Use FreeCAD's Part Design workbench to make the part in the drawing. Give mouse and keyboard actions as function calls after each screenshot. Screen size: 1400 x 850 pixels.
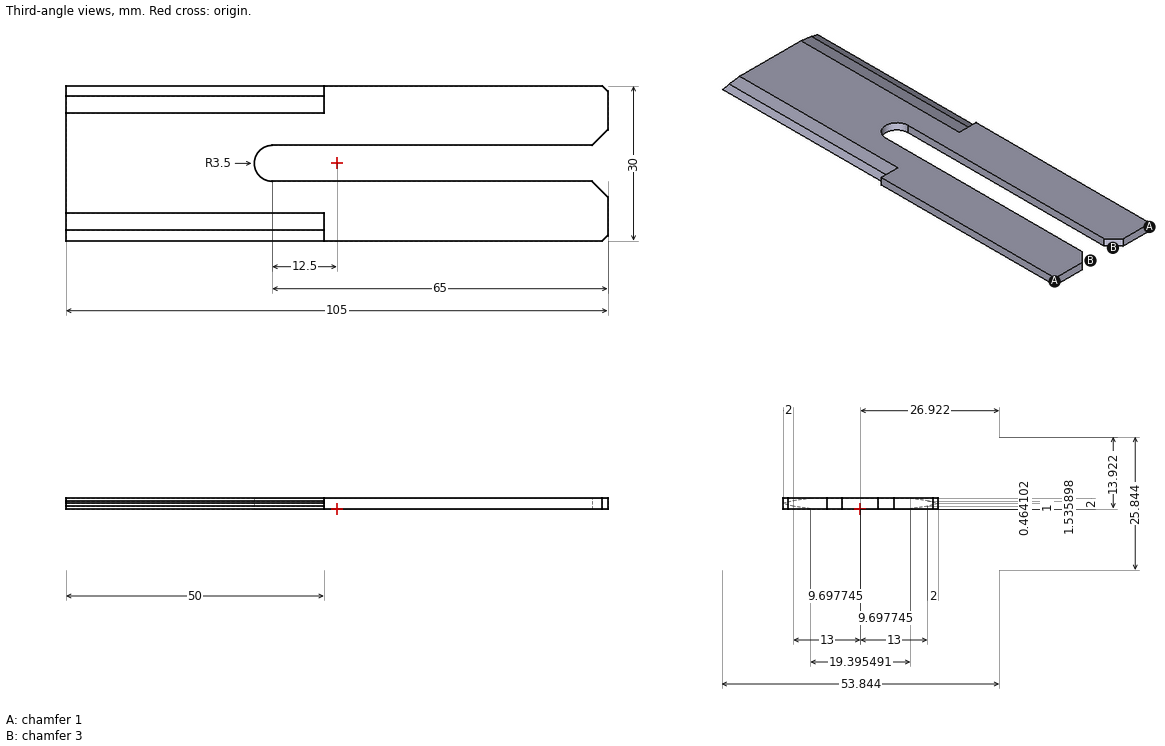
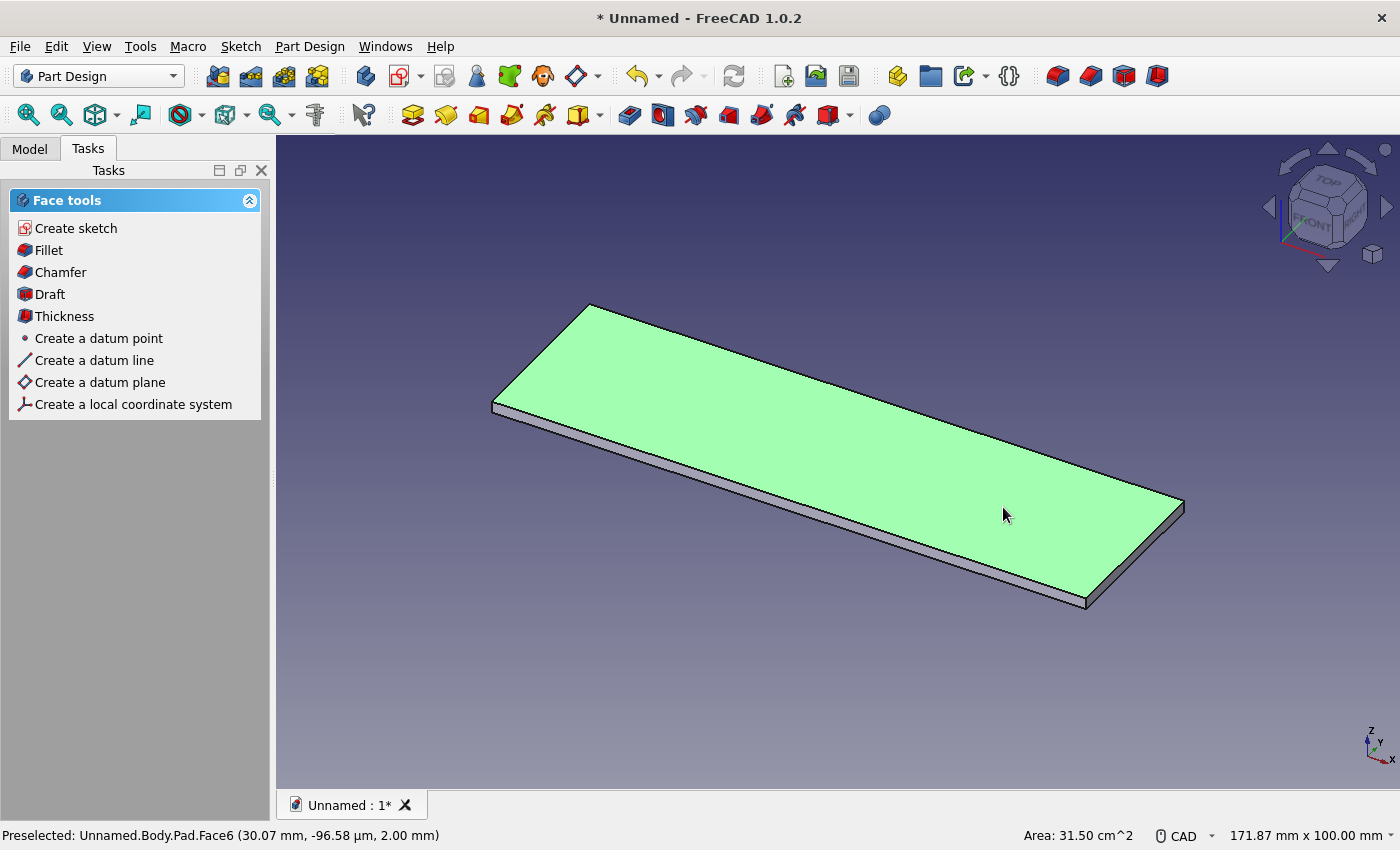
click(398, 76)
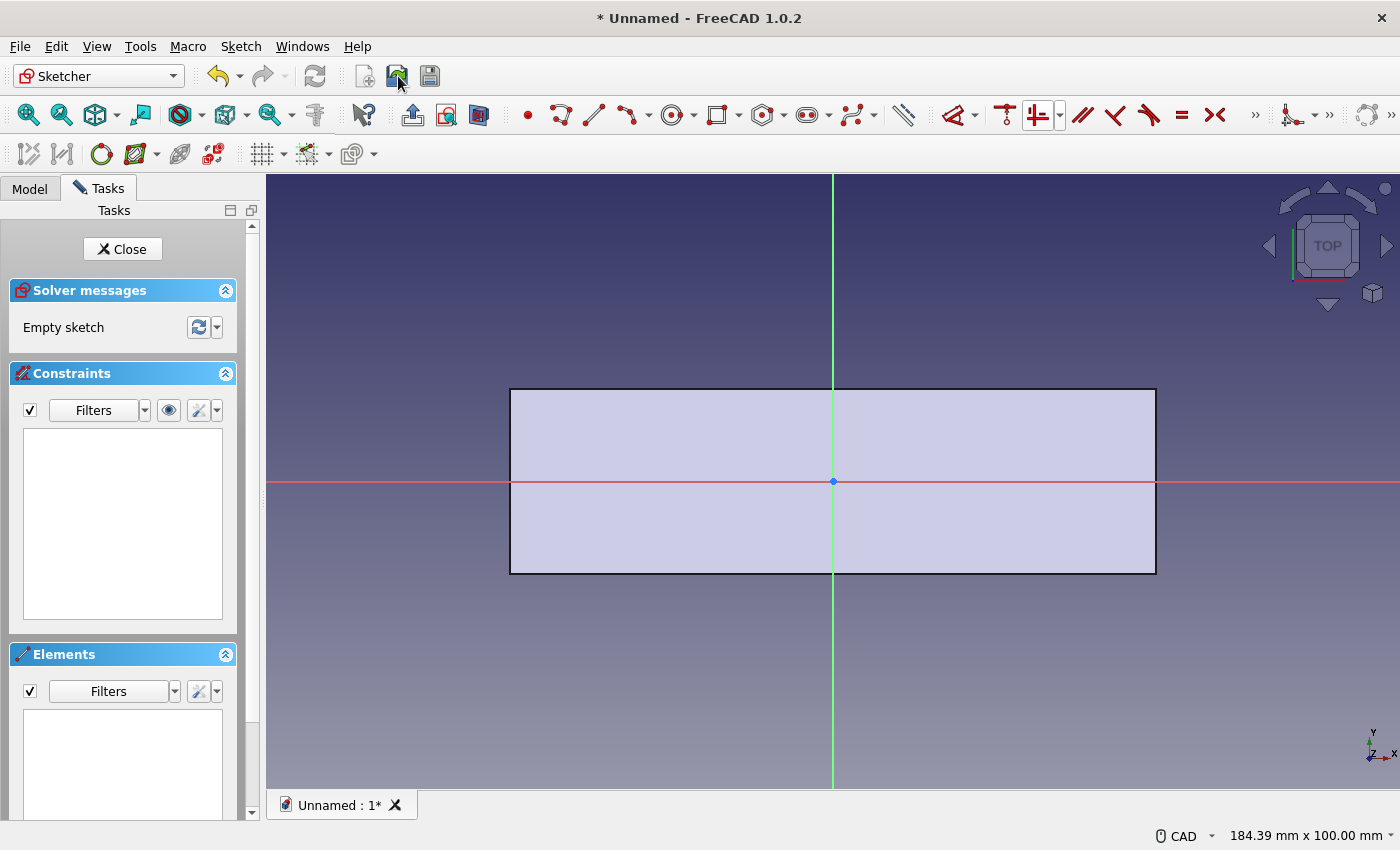
scroll(1235, 482, up, 2)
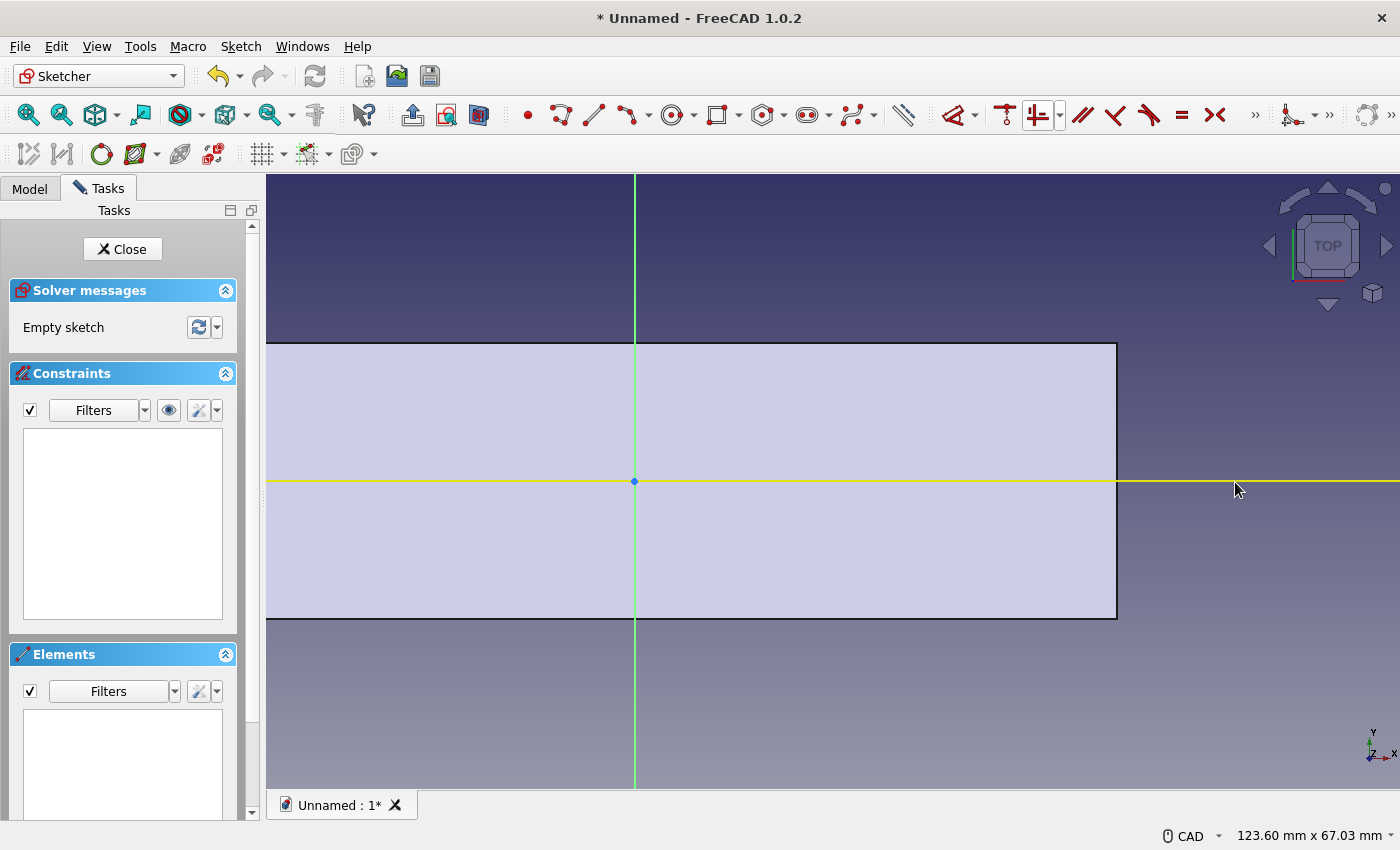
click(561, 116)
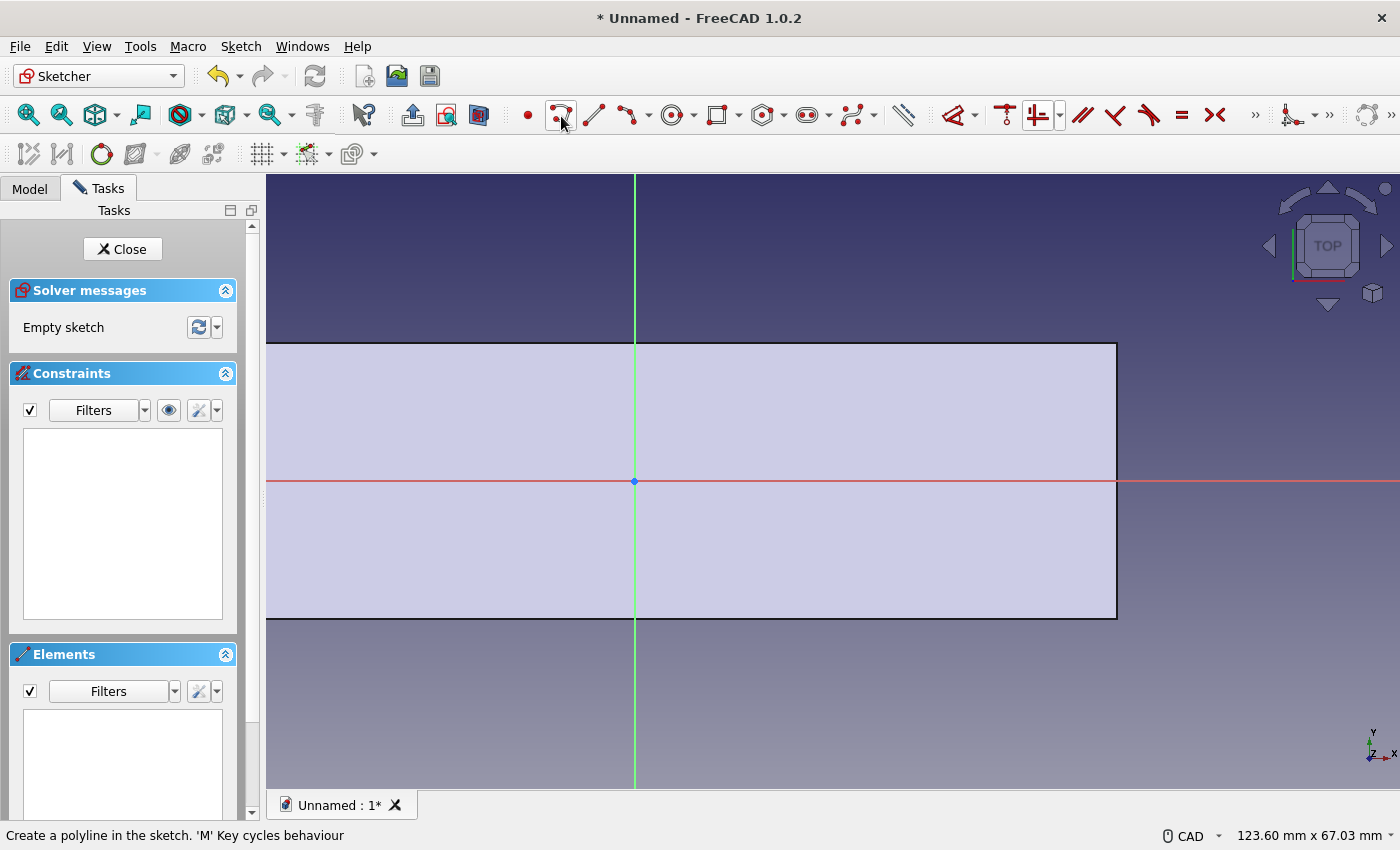
click(520, 513)
click(1117, 513)
click(1117, 449)
click(520, 449)
right_click(520, 449)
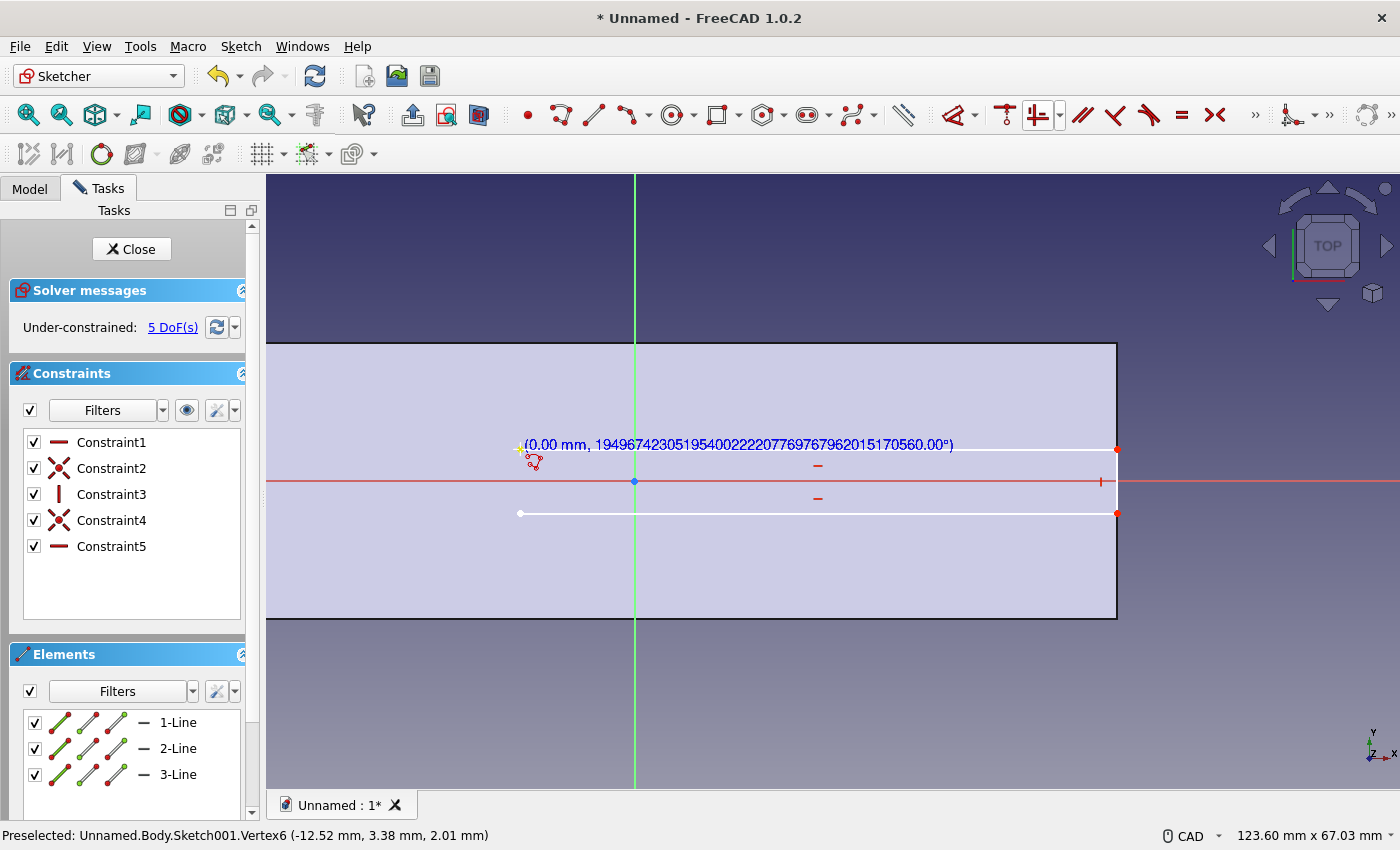
click(626, 116)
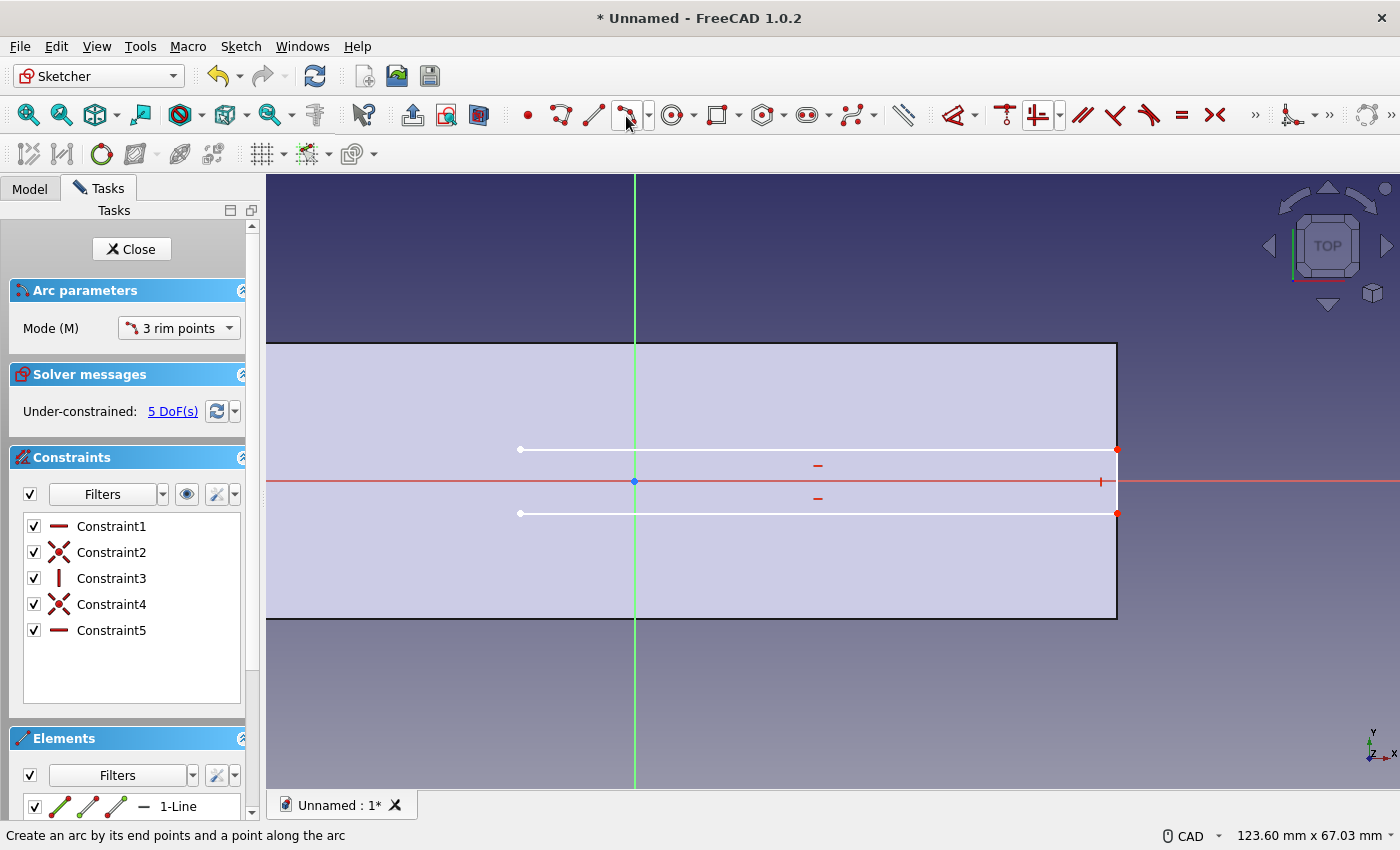
click(520, 450)
click(520, 514)
click(494, 462)
key(Escape)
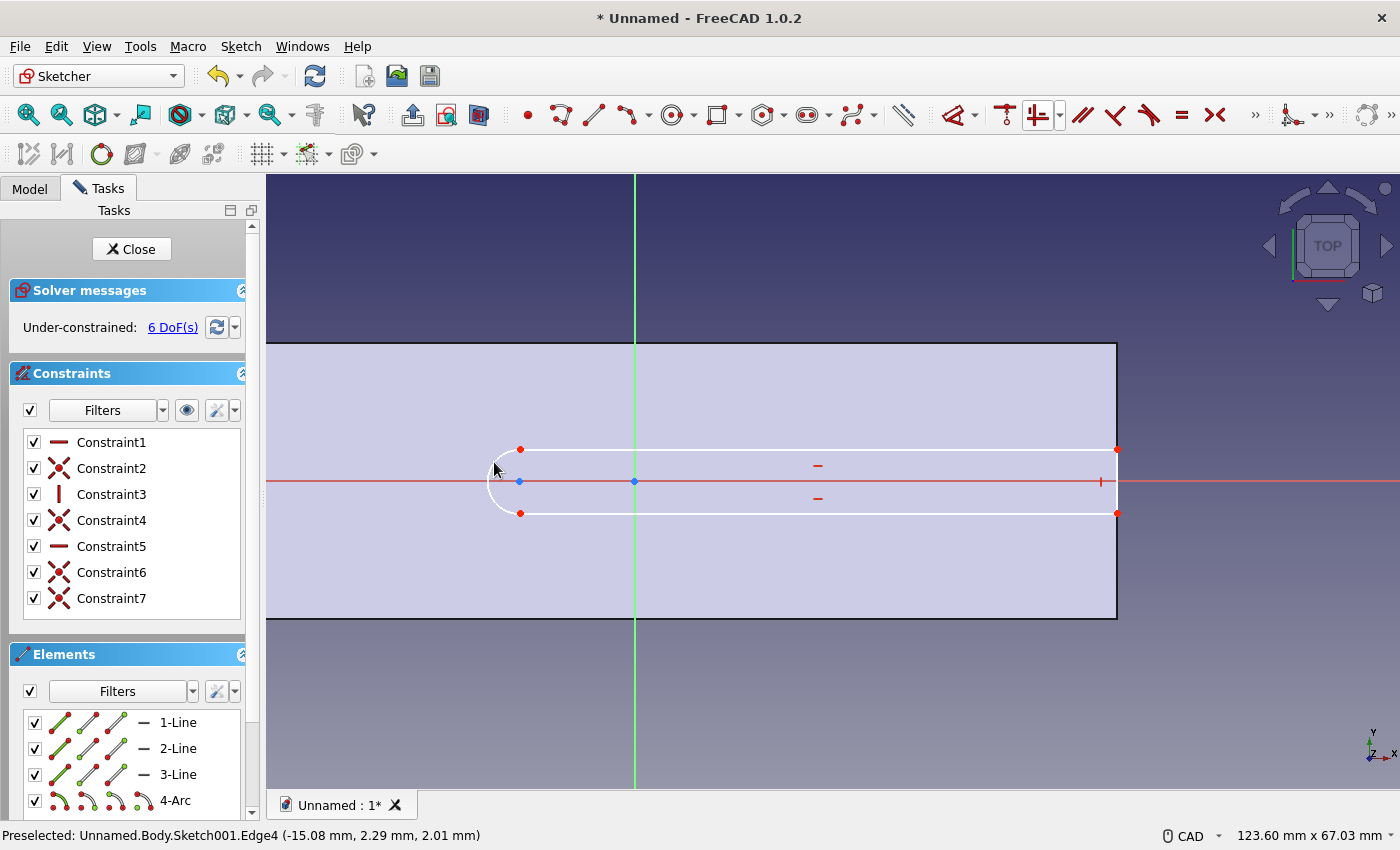
click(699, 514)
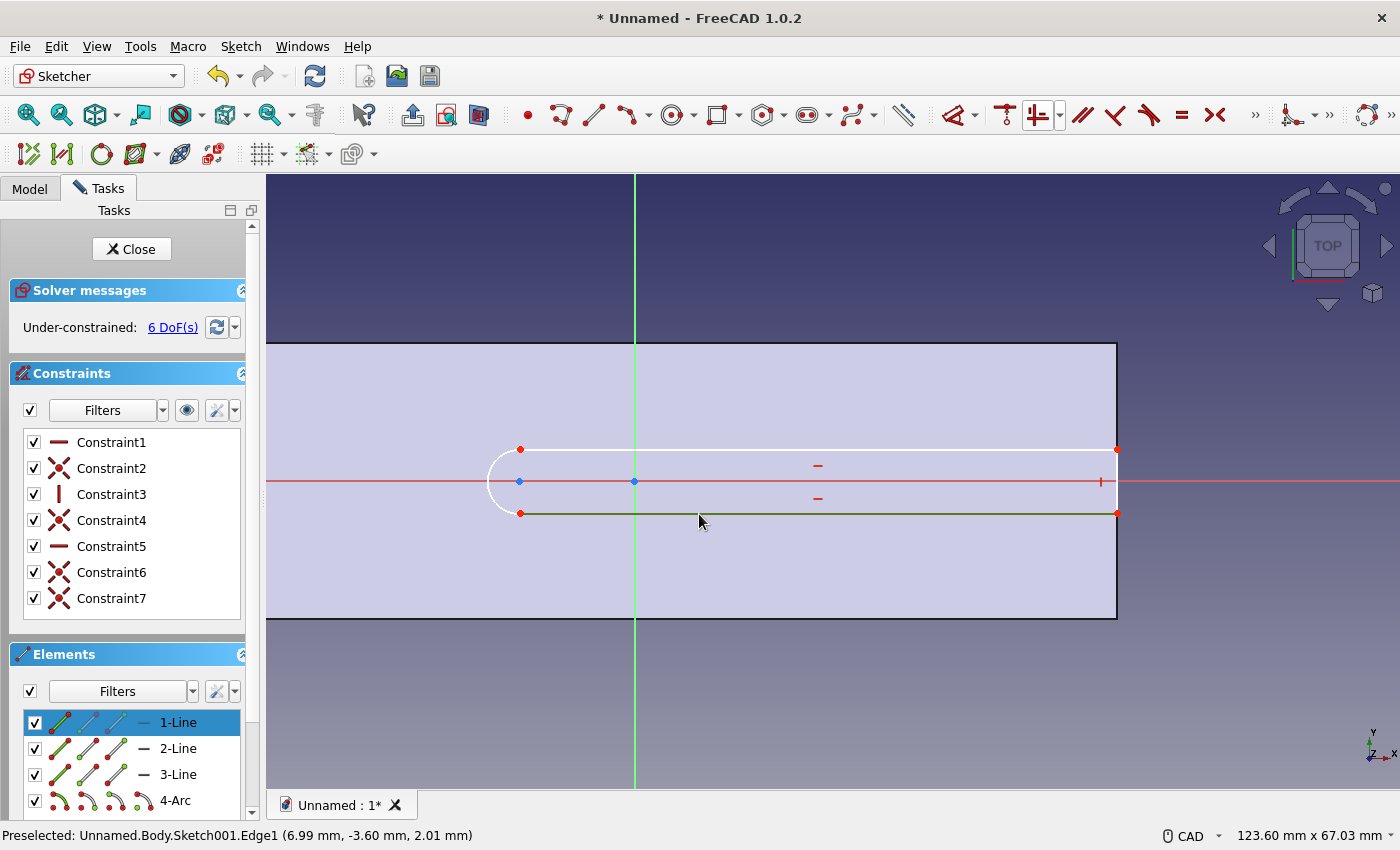
click(494, 463)